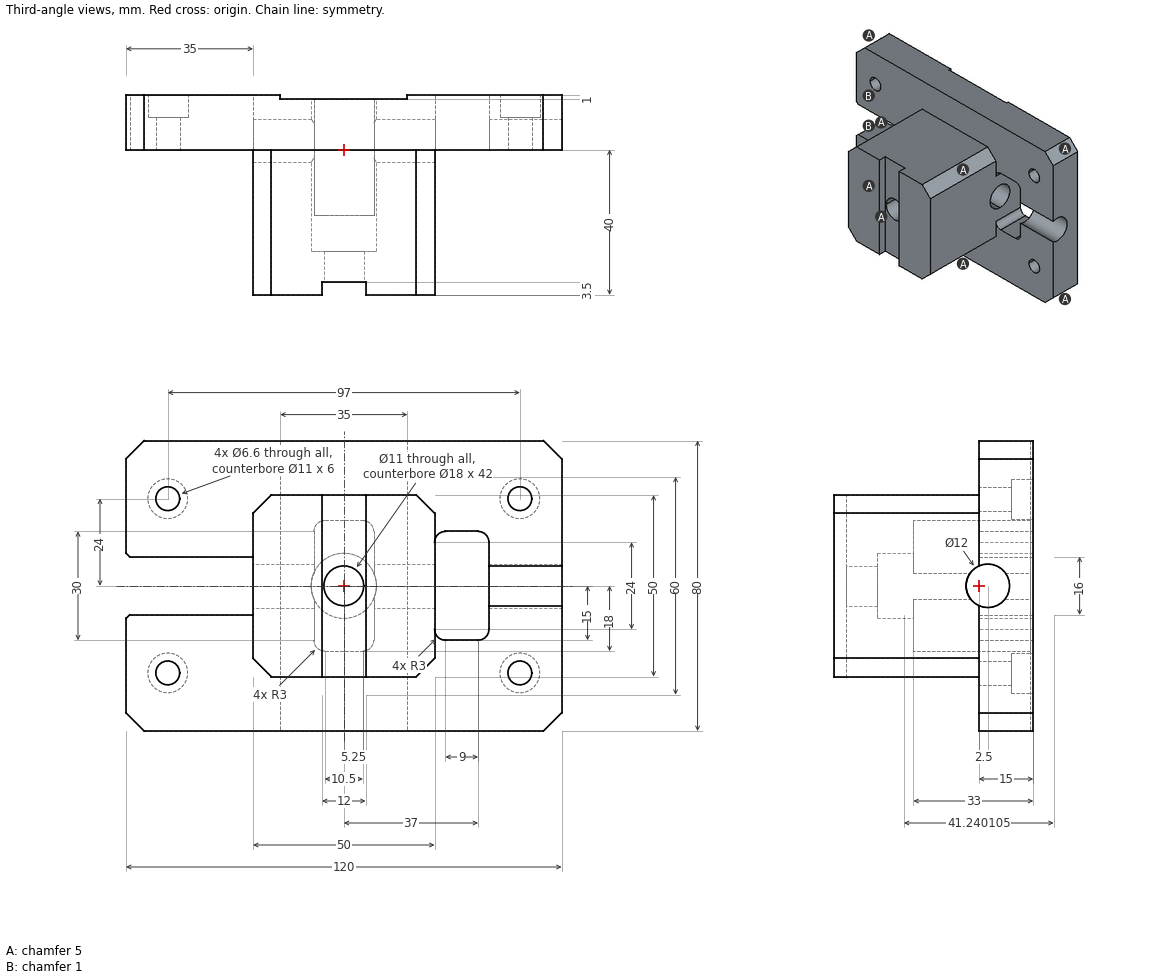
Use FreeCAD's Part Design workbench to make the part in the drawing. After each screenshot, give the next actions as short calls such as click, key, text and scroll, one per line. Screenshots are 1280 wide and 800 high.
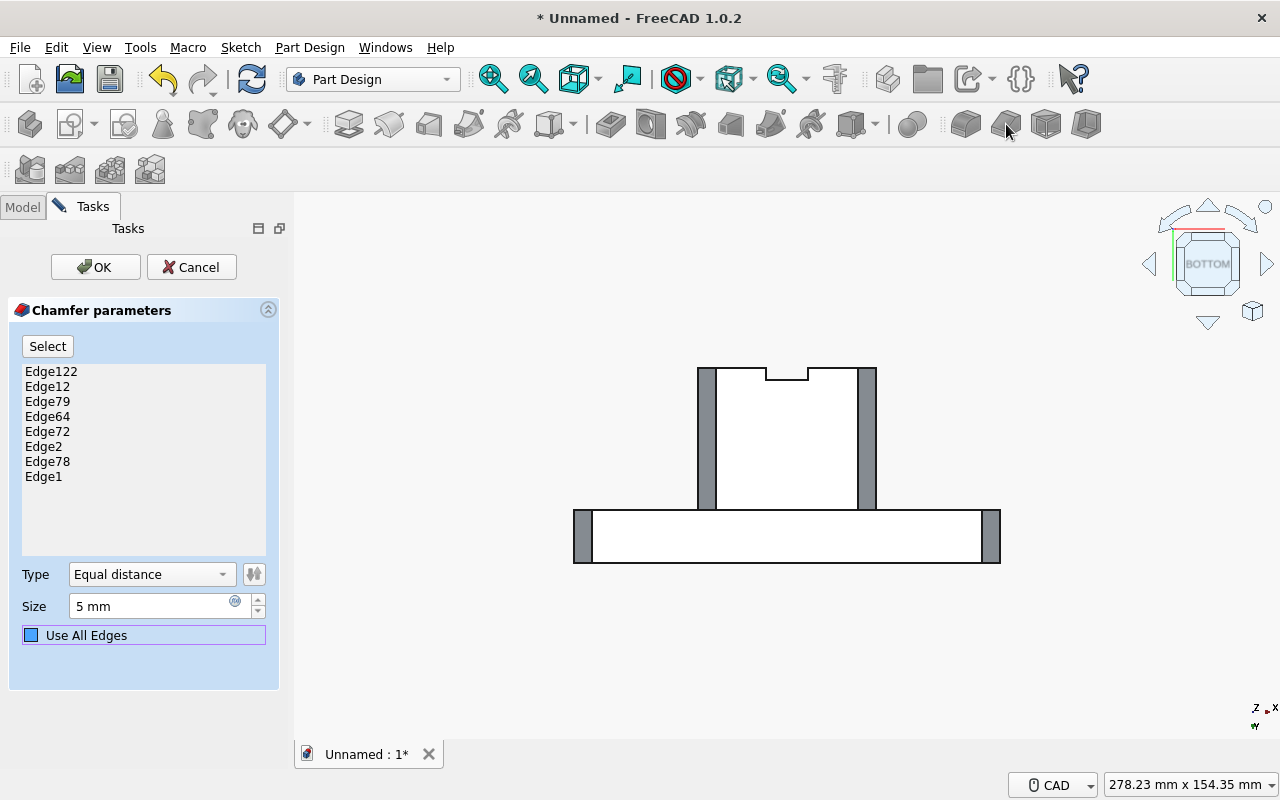
click(96, 267)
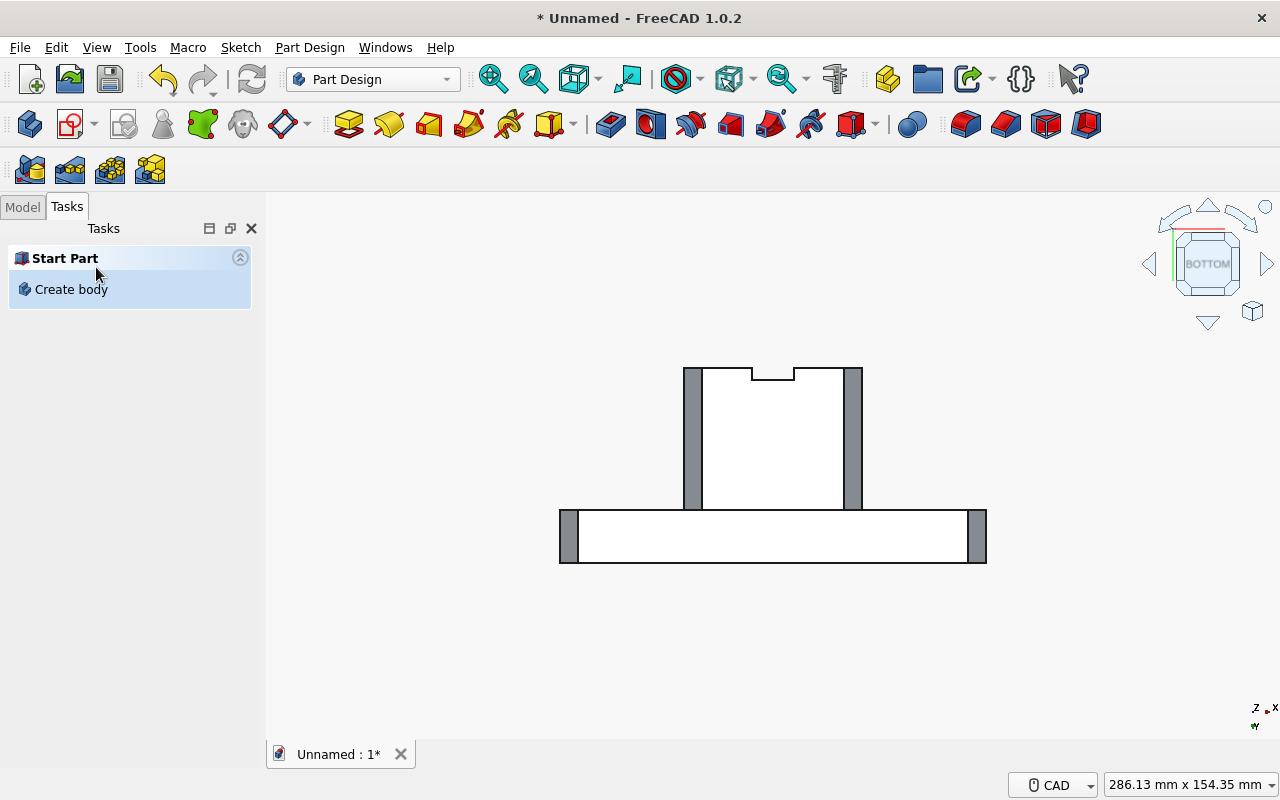
click(494, 80)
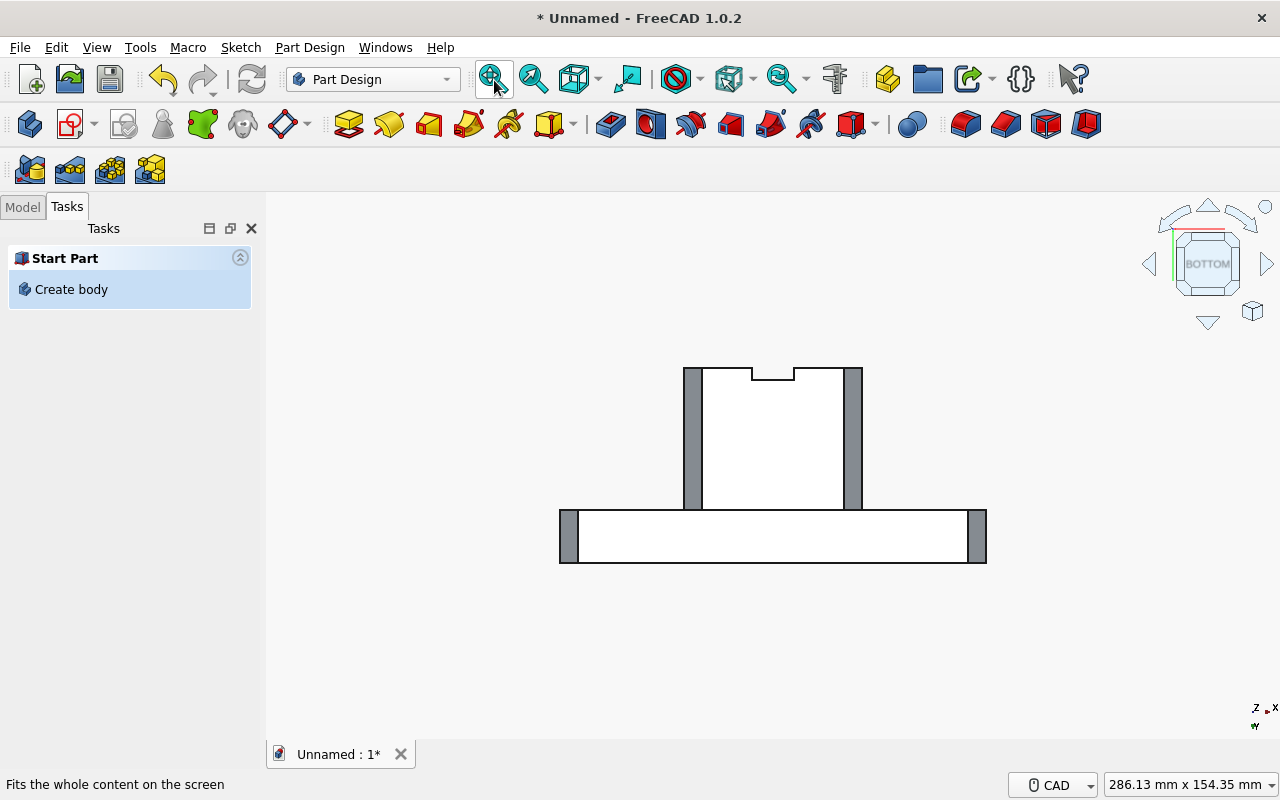
key(0)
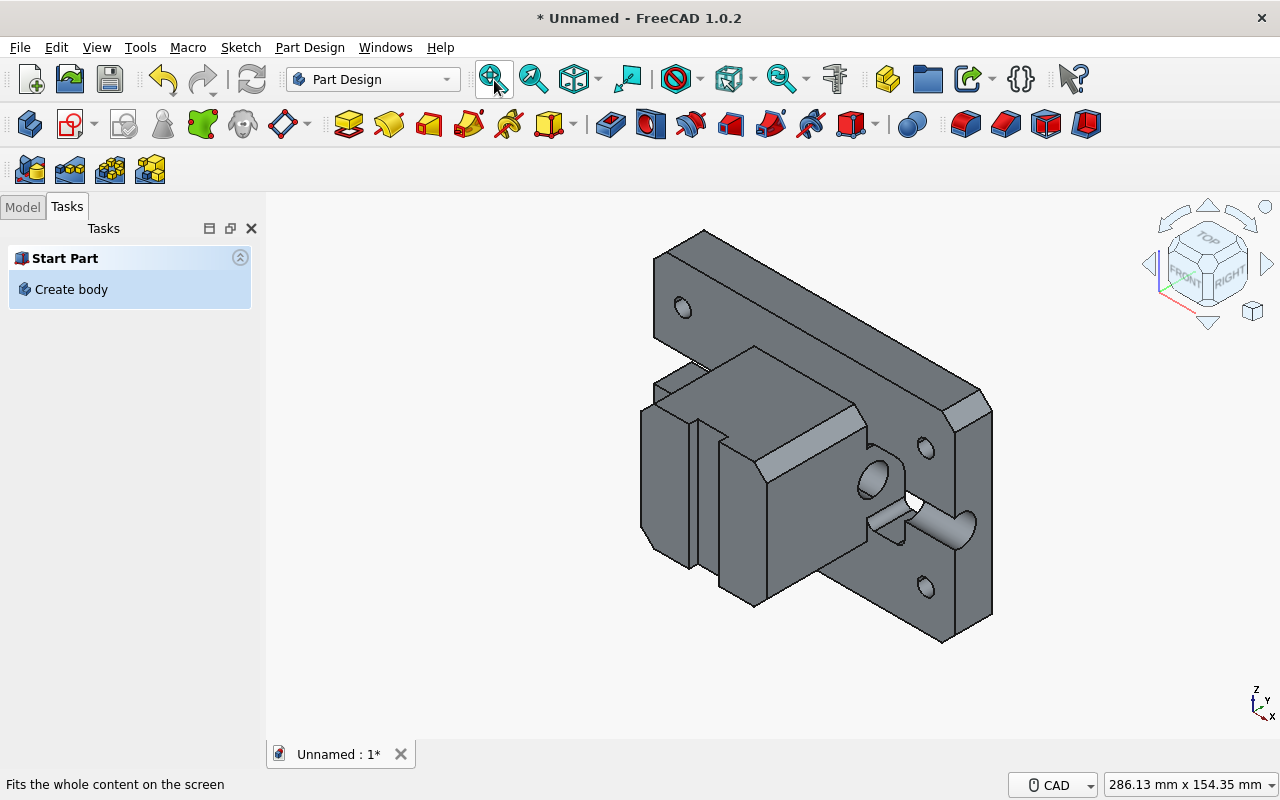
key(2)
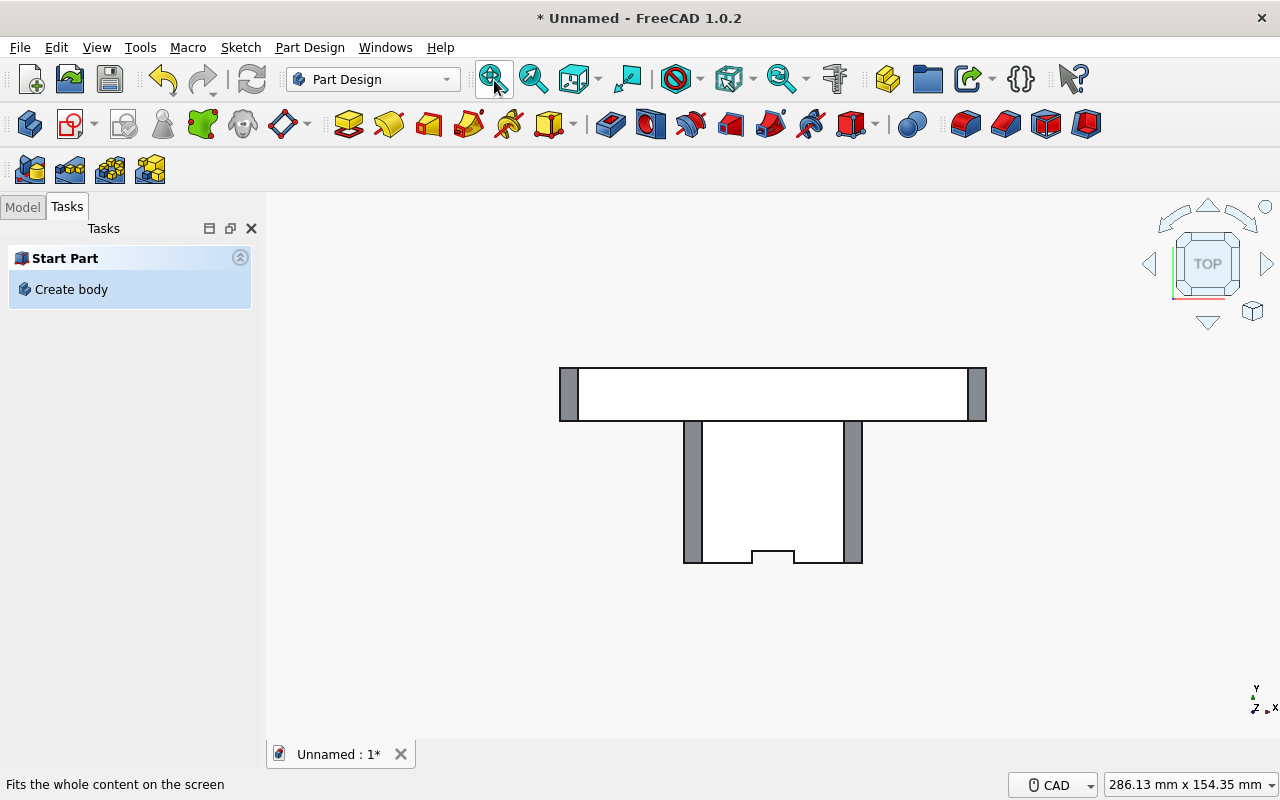
click(494, 80)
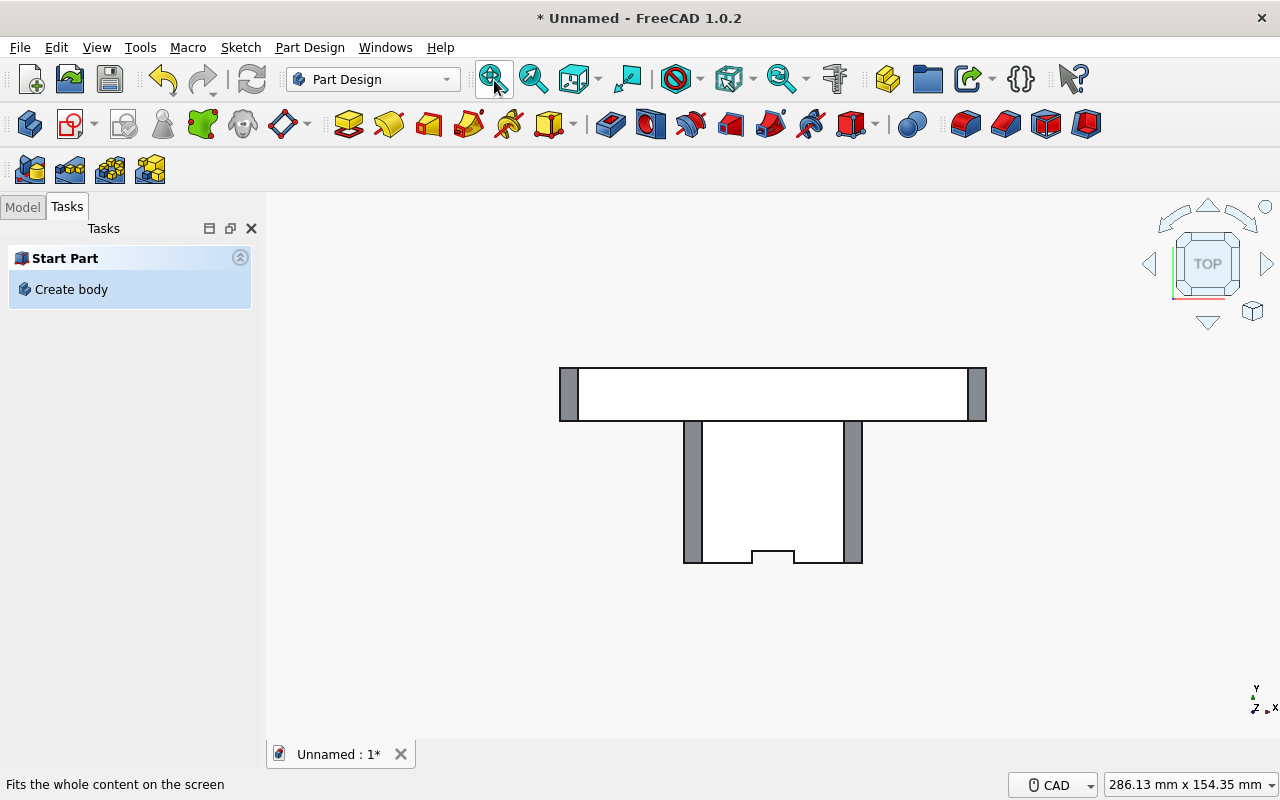
key(1)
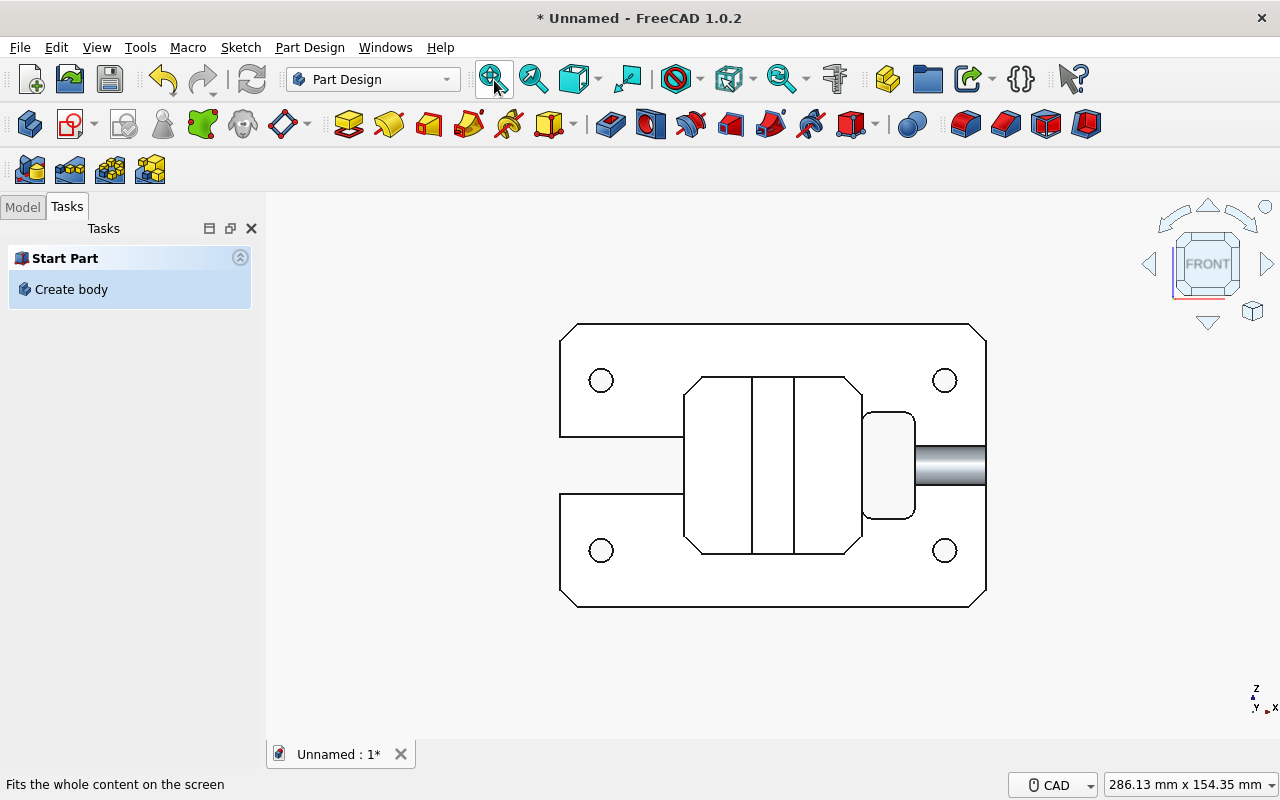
key(3)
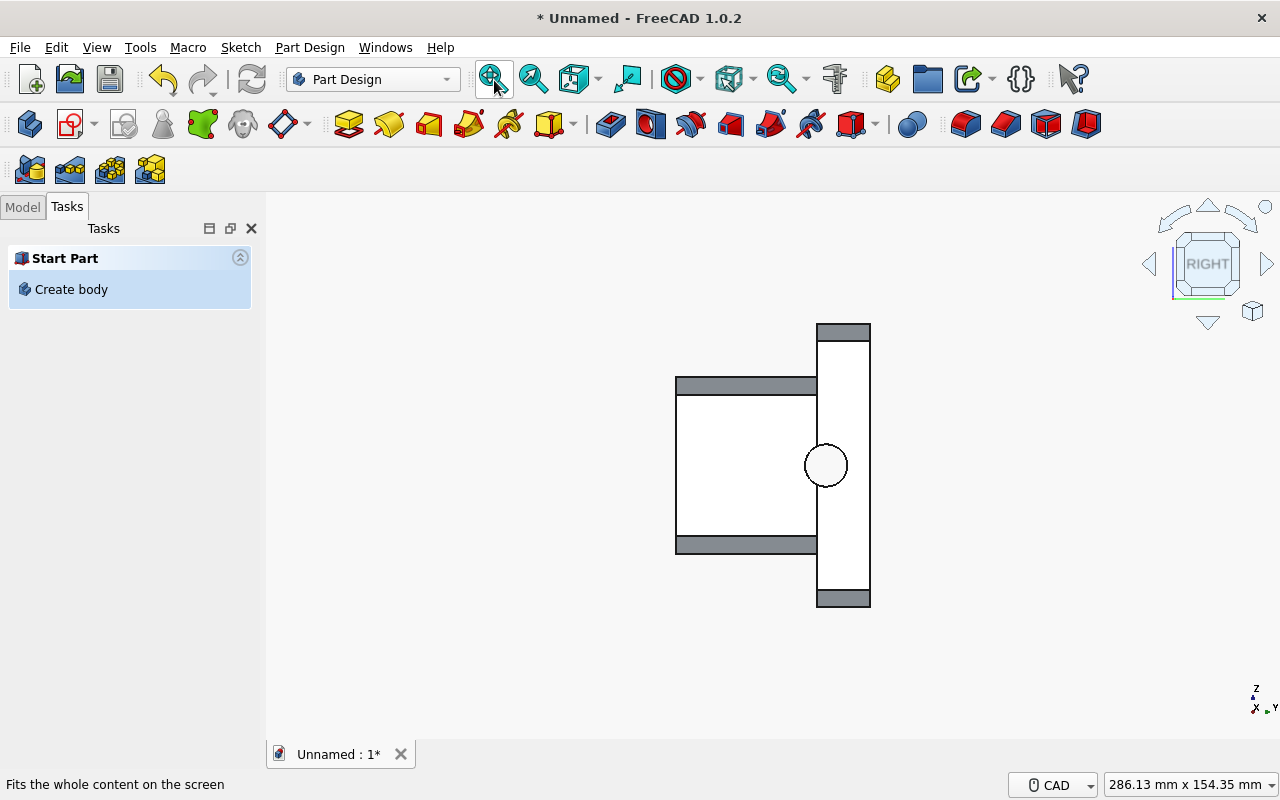
key(5)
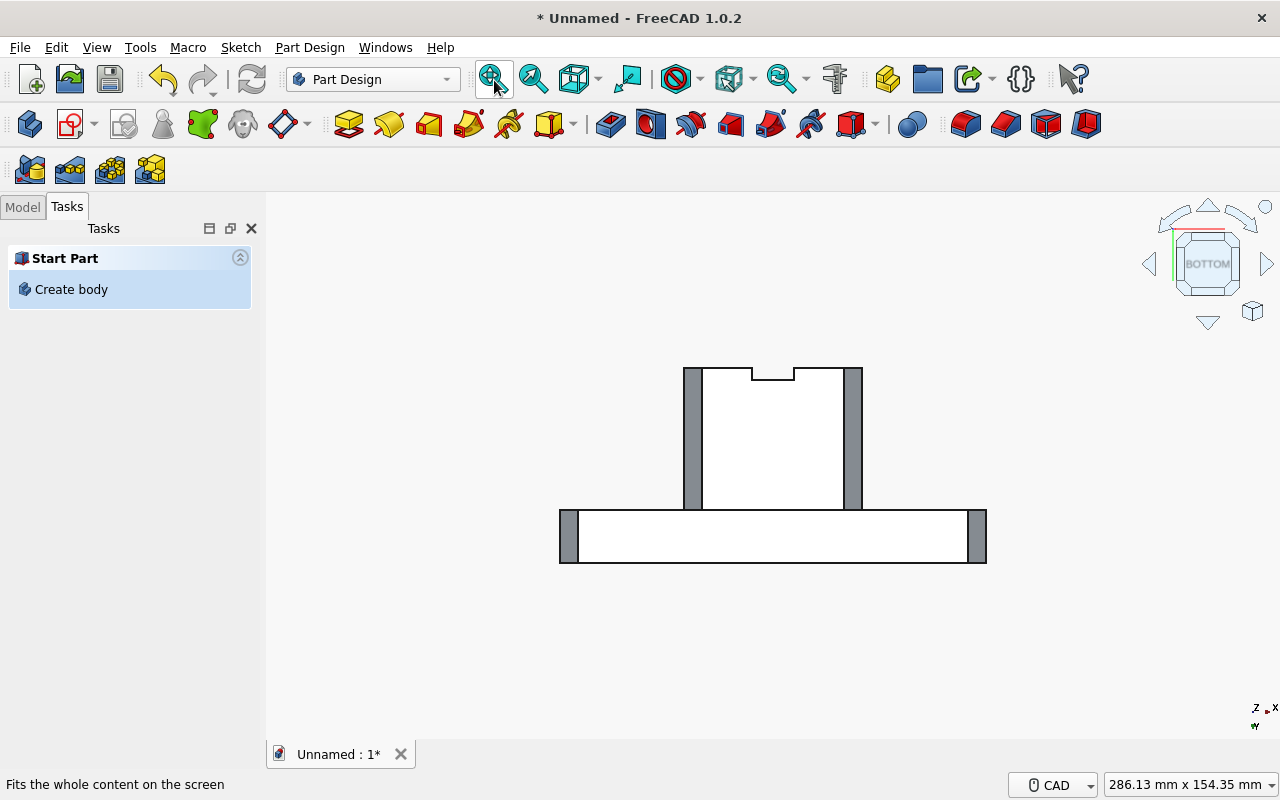
key(v)
key(f)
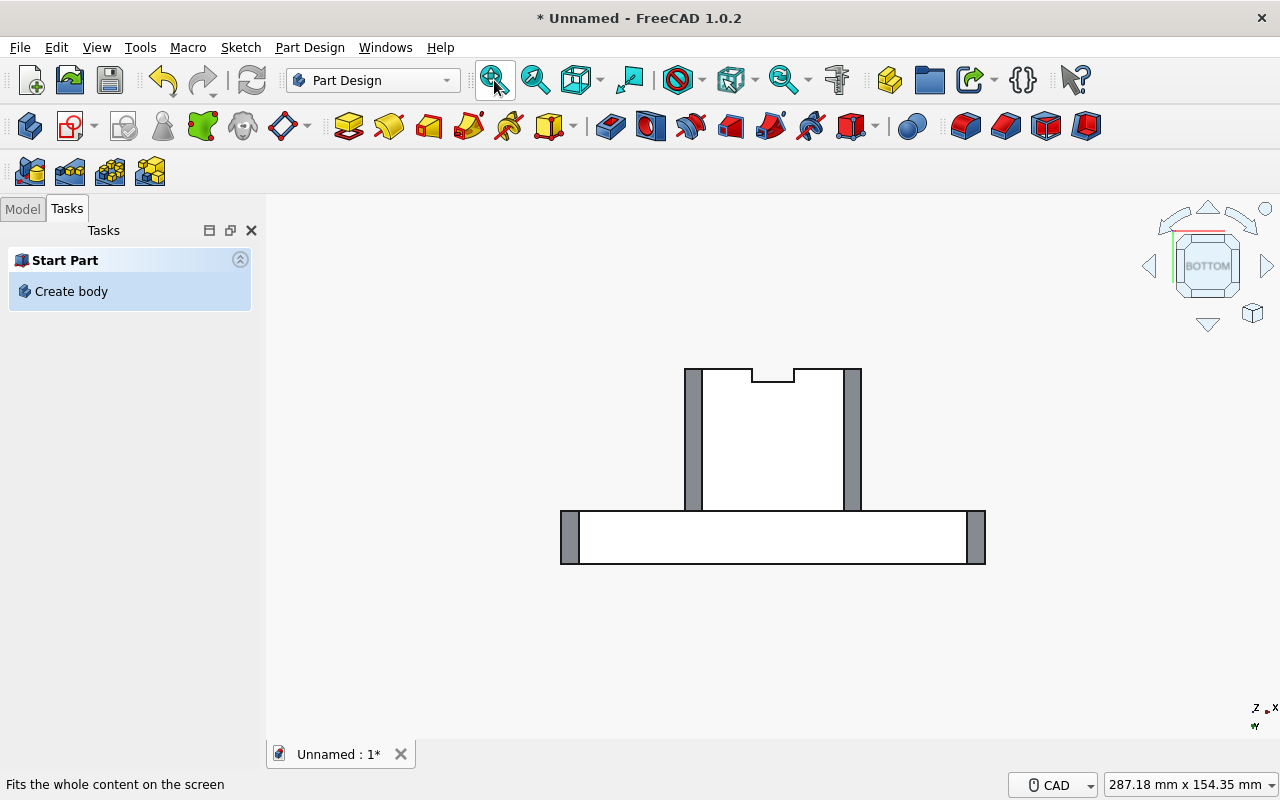
key(4)